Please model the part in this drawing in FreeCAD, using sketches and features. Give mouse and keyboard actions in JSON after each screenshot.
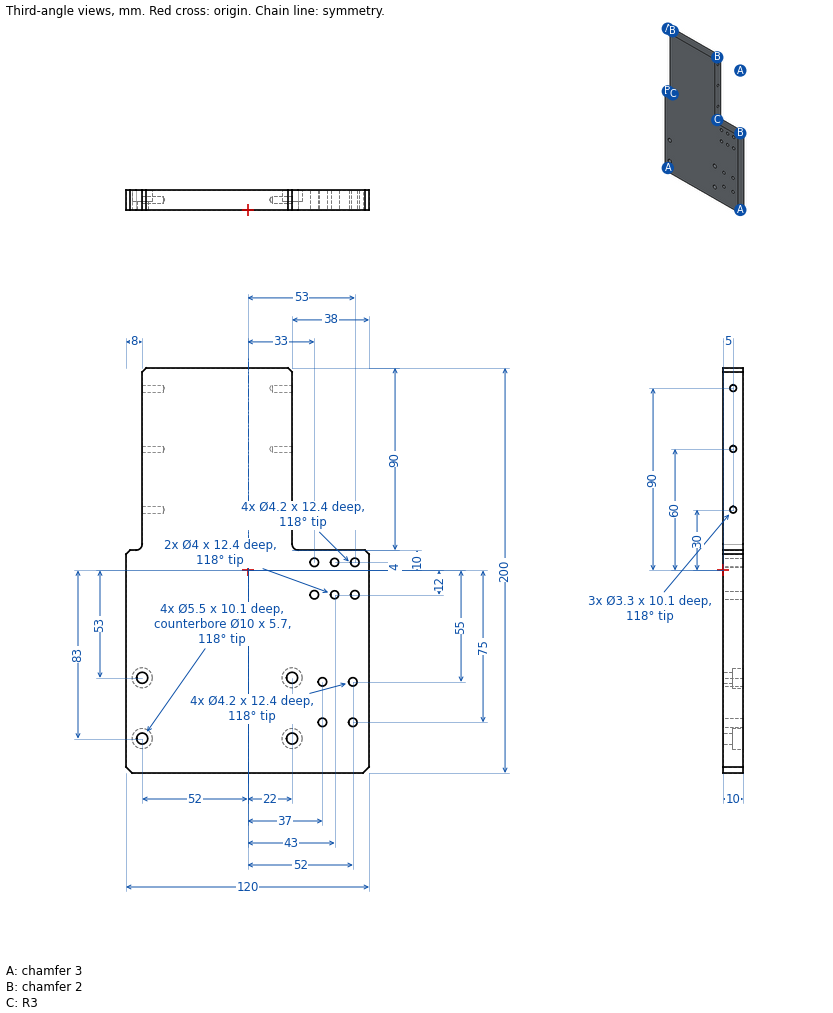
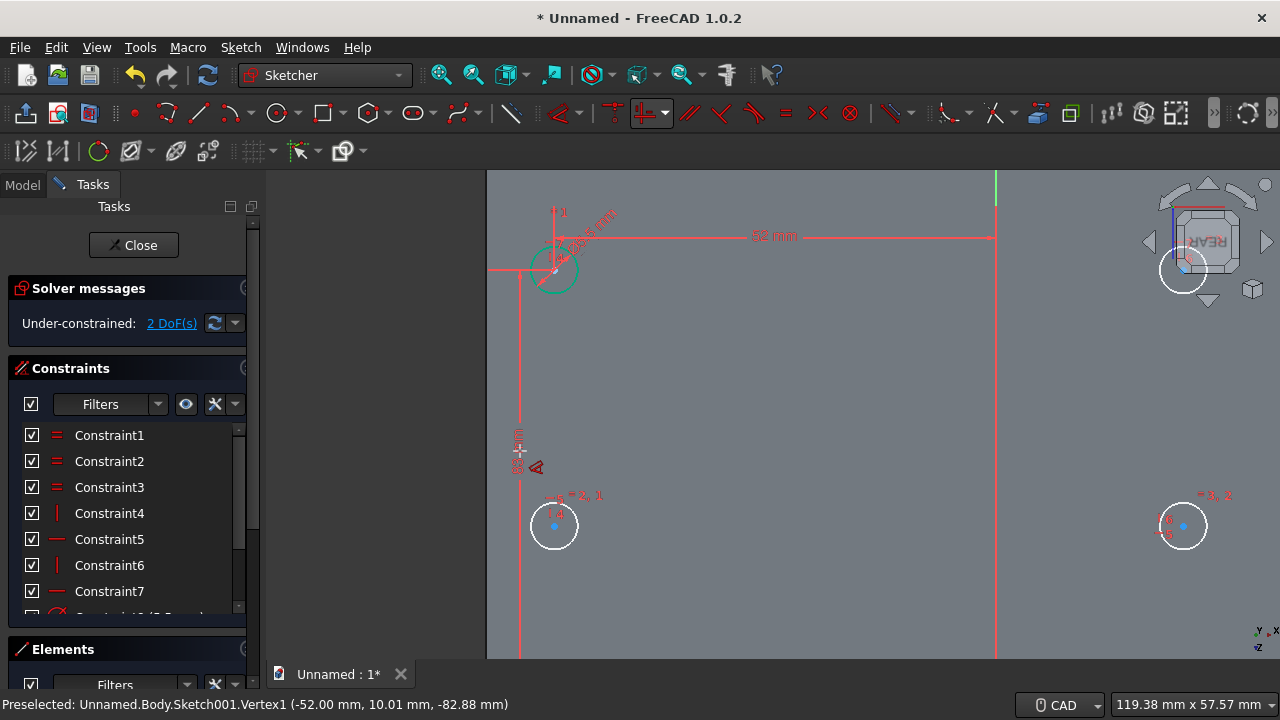
{"action": "left_click", "coordinate": [554, 526]}
{"action": "left_click", "coordinate": [520, 579]}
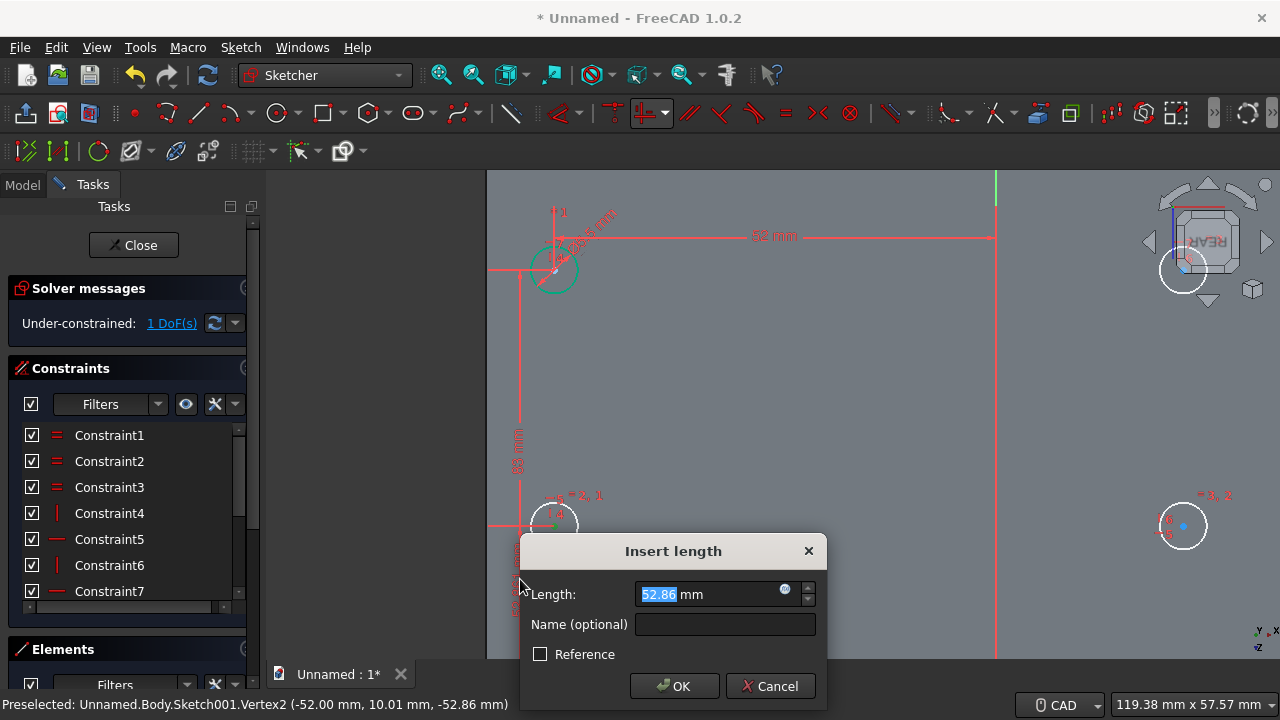
{"action": "type", "text": "53"}
{"action": "key", "text": "Return"}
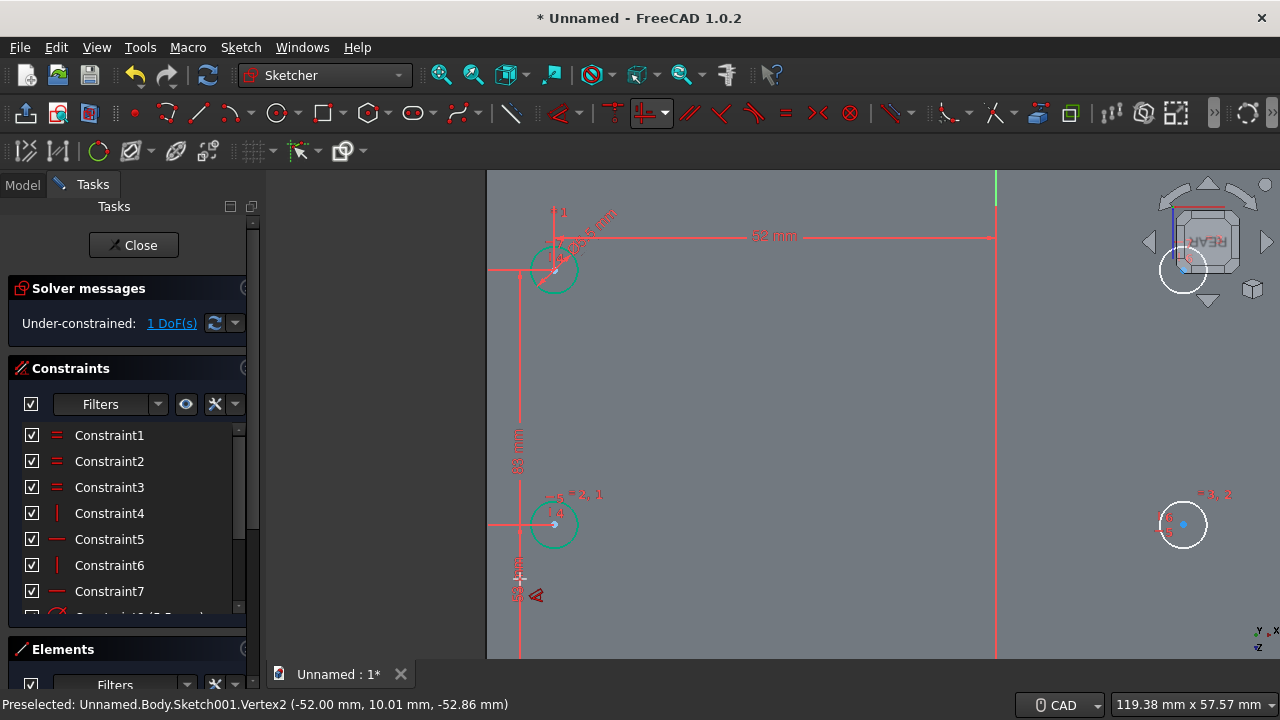
{"action": "scroll", "coordinate": [571, 254], "scroll_direction": "down", "scroll_amount": 4}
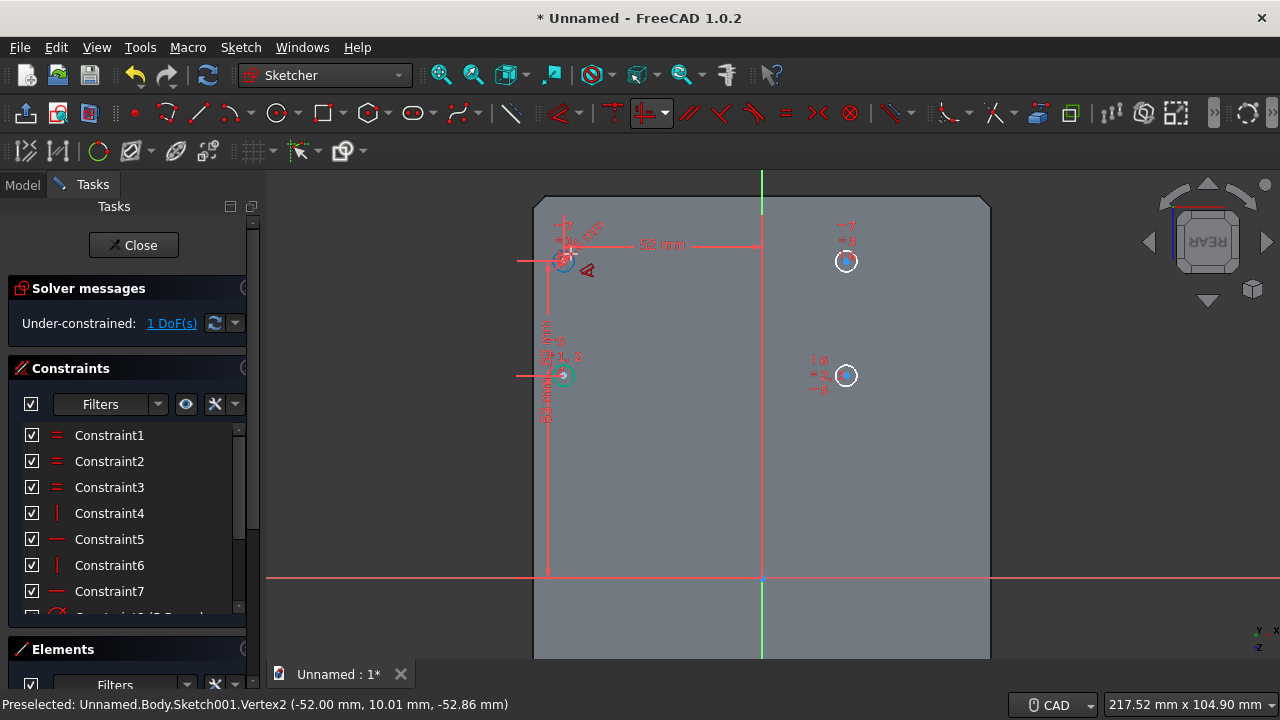
{"action": "left_click", "coordinate": [846, 376]}
{"action": "left_click", "coordinate": [804, 612]}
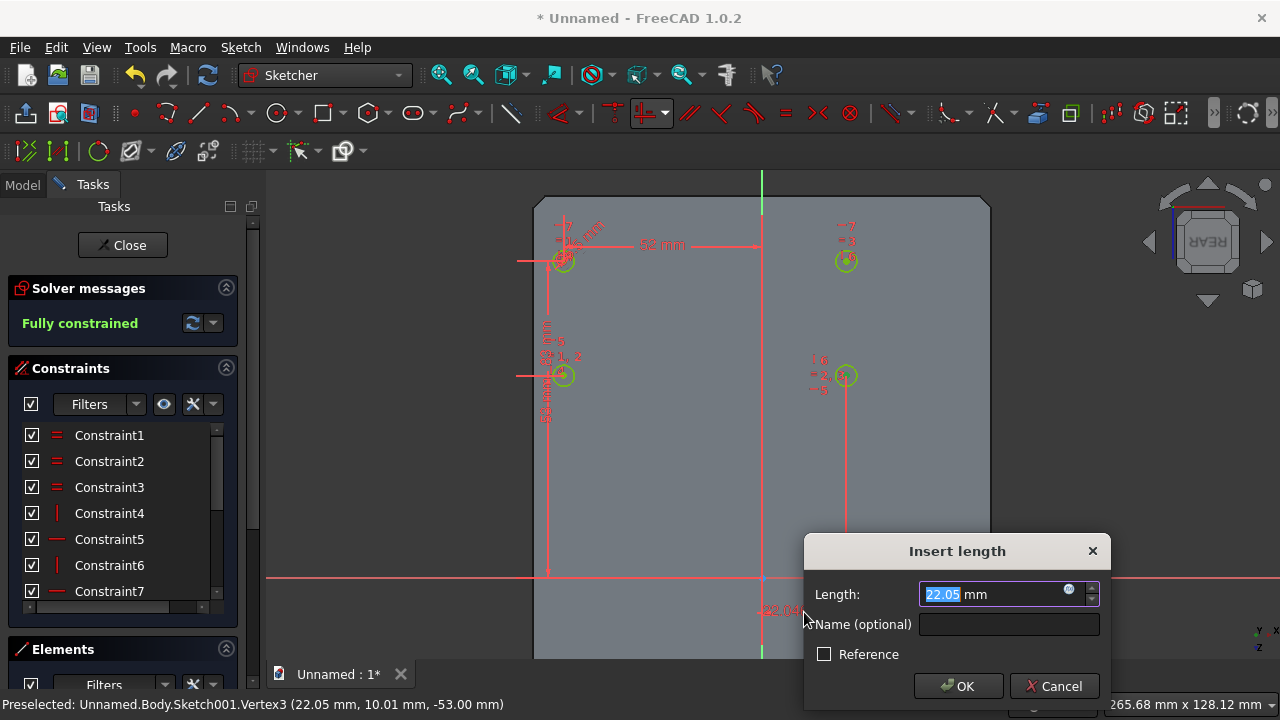
{"action": "type", "text": "22"}
{"action": "key", "text": "Return"}
{"action": "key", "text": "Escape"}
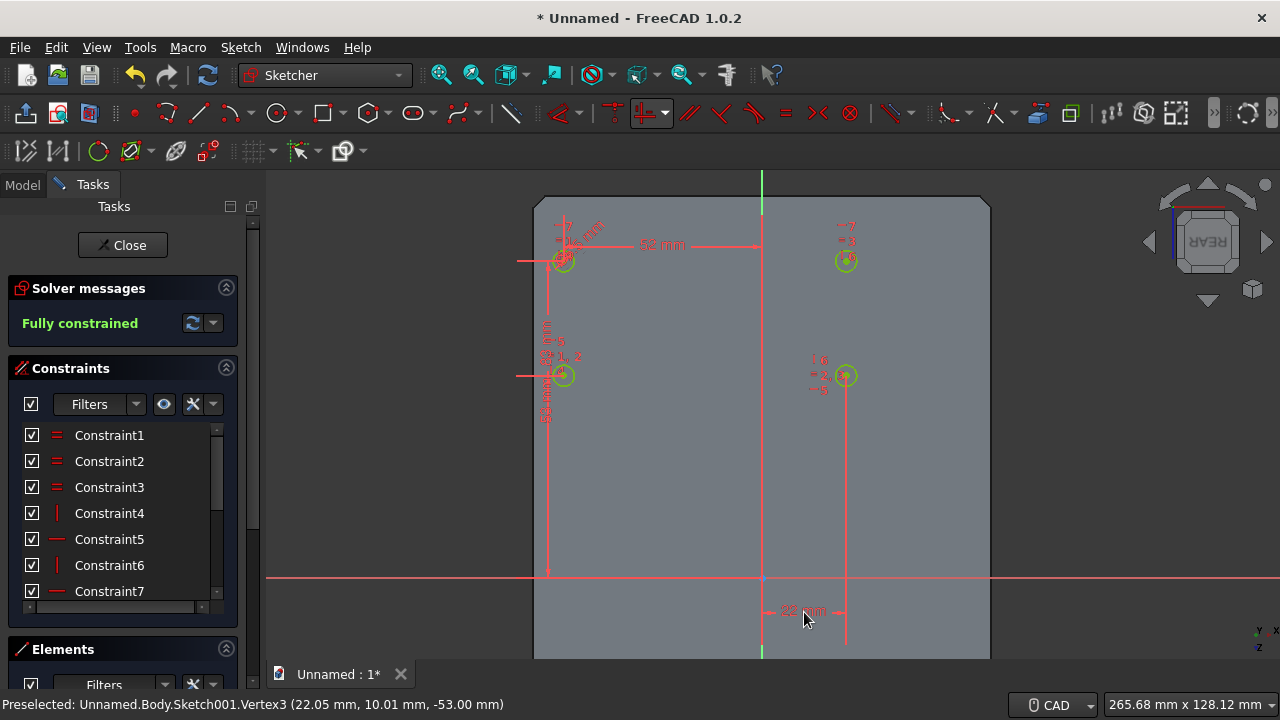
{"action": "left_click", "coordinate": [123, 245]}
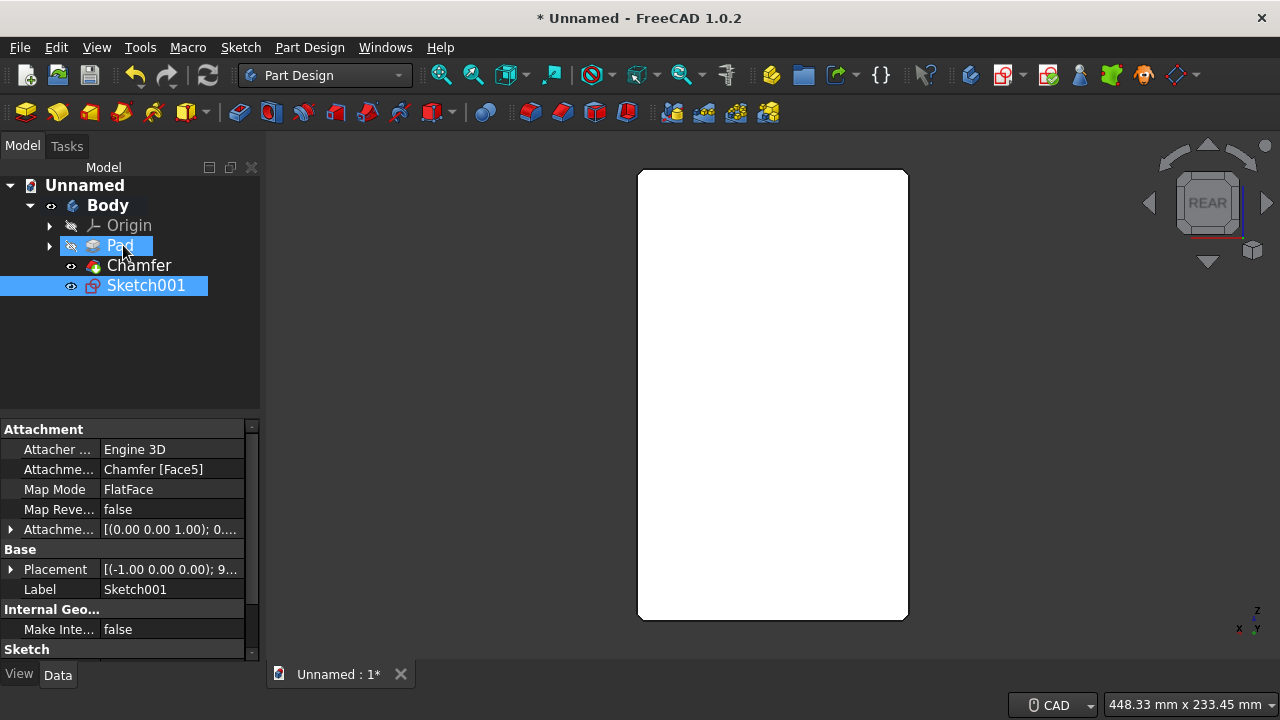
{"action": "left_click", "coordinate": [272, 112]}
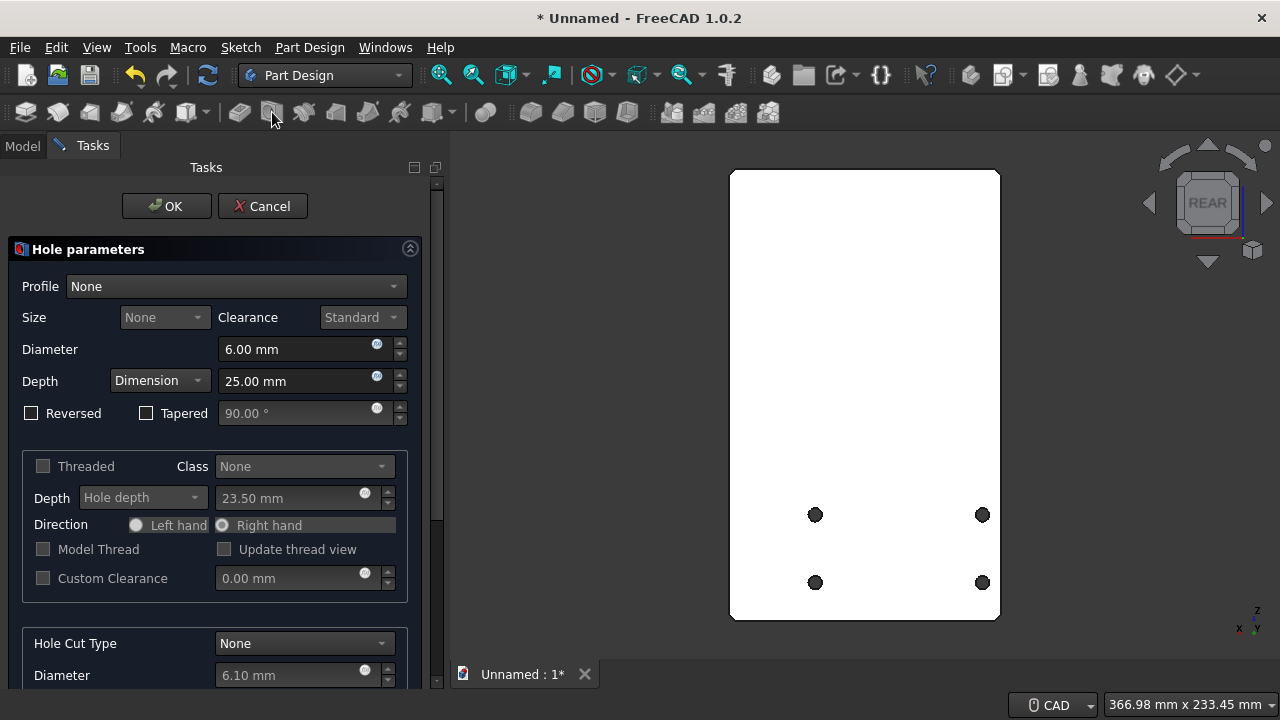
{"action": "triple_click", "coordinate": [305, 349]}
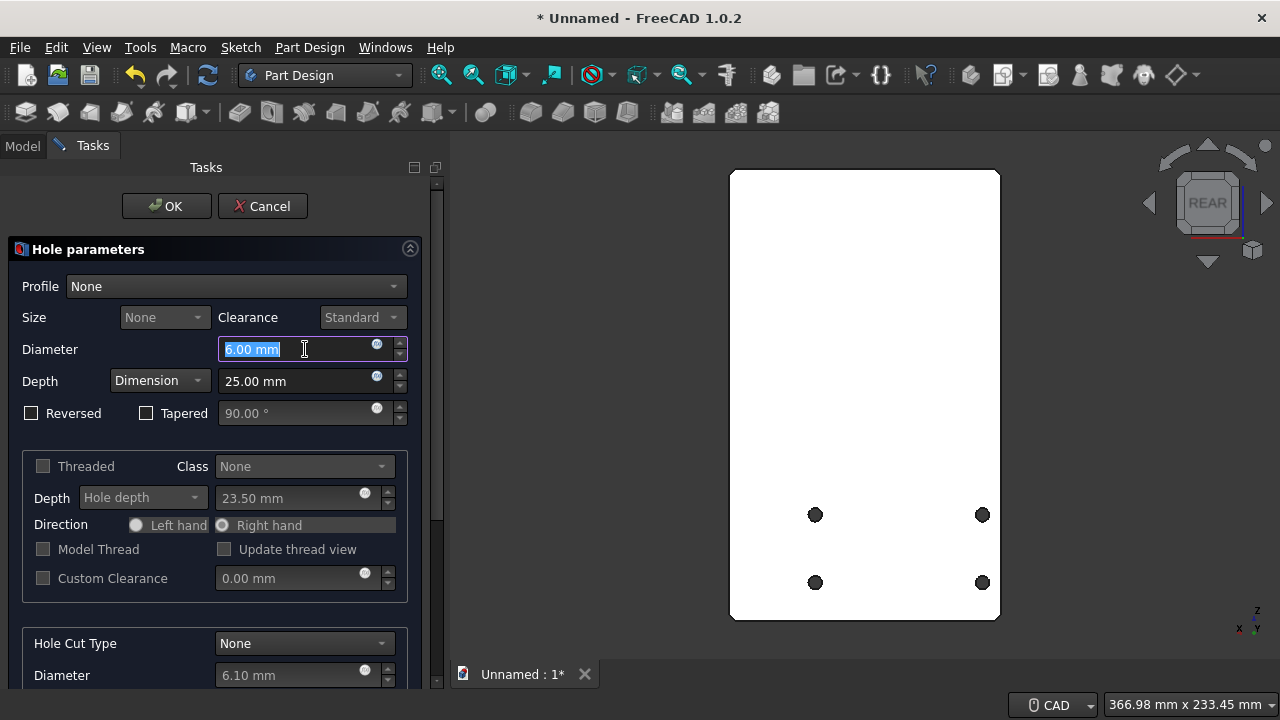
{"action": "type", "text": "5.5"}
{"action": "key", "text": "Tab"}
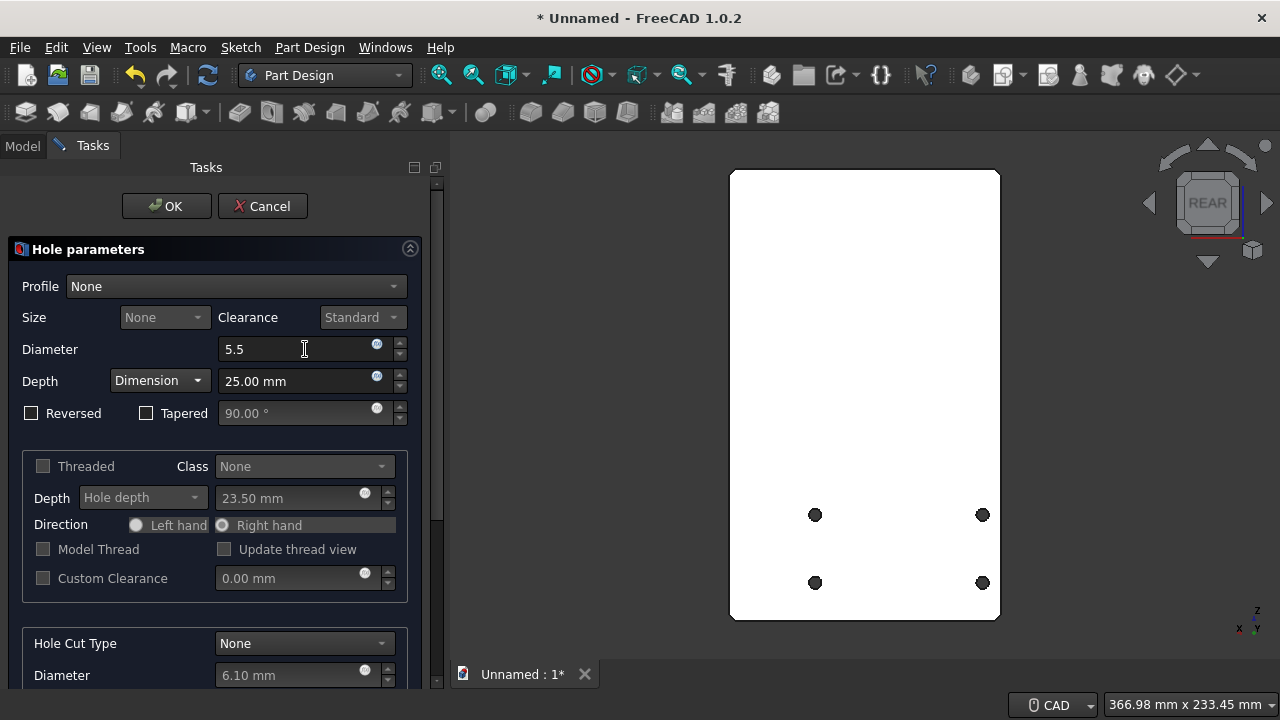
{"action": "triple_click", "coordinate": [305, 381]}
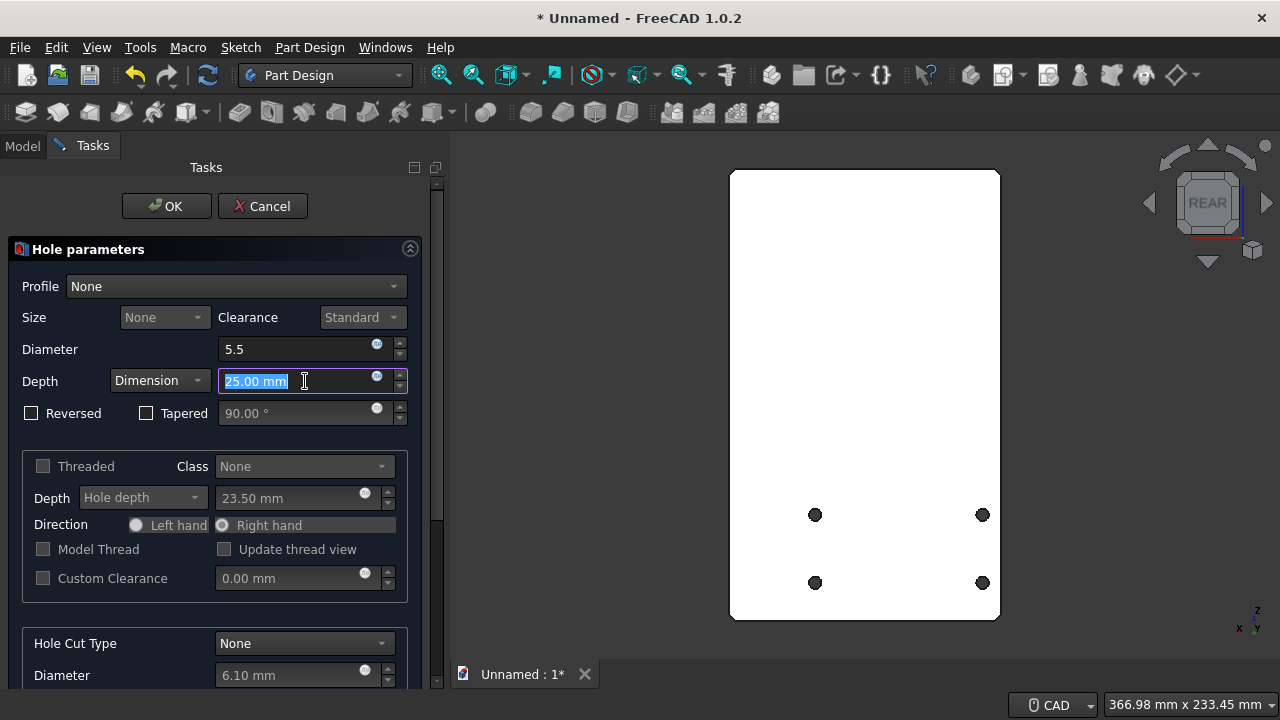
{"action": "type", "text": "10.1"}
{"action": "key", "text": "Tab"}